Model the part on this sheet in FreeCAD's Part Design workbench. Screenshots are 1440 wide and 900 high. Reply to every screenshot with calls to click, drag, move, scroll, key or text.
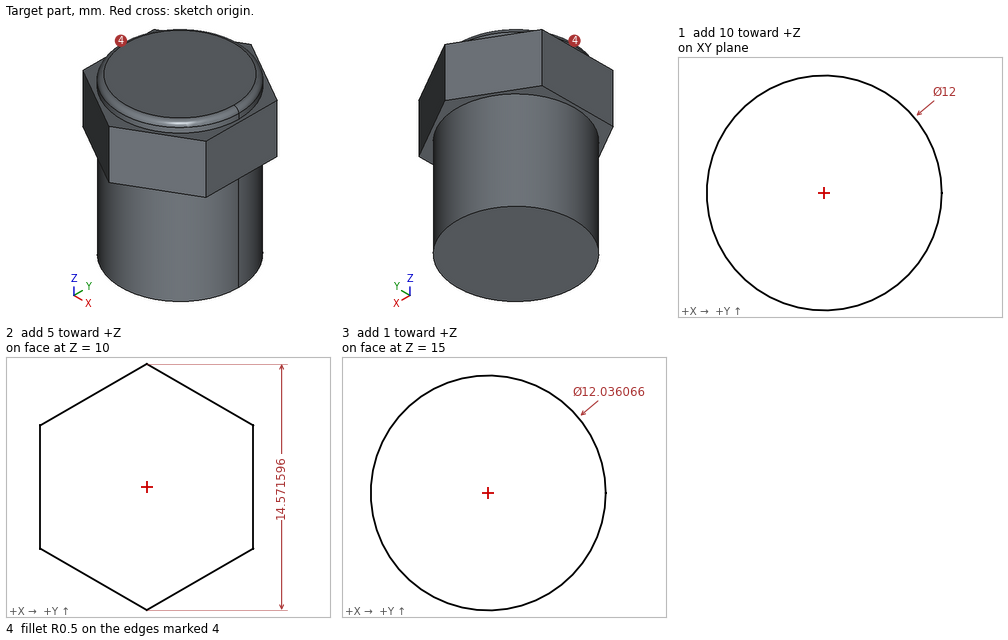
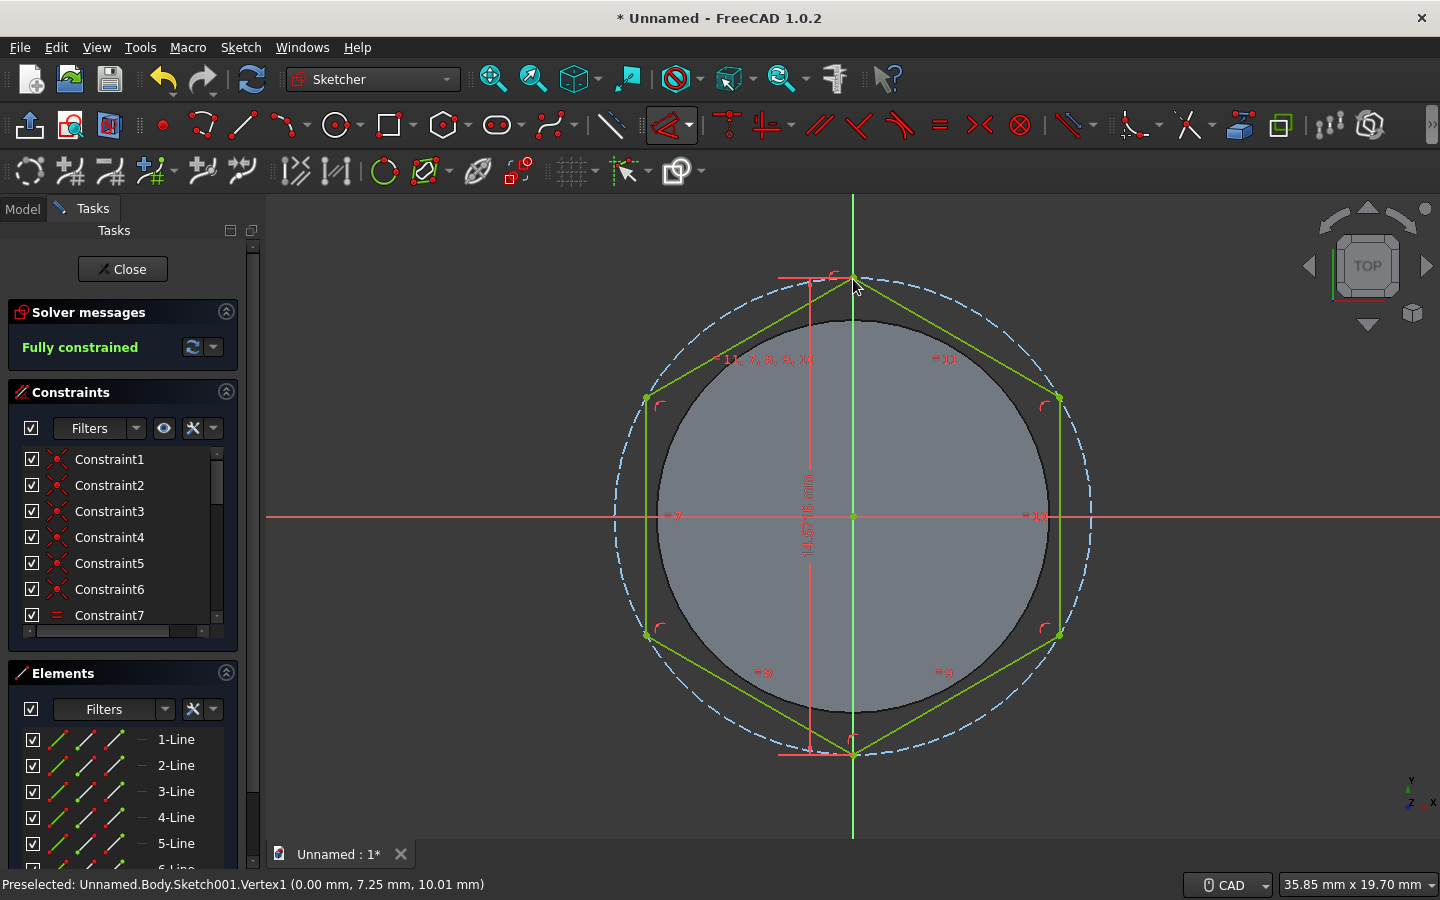
click(123, 269)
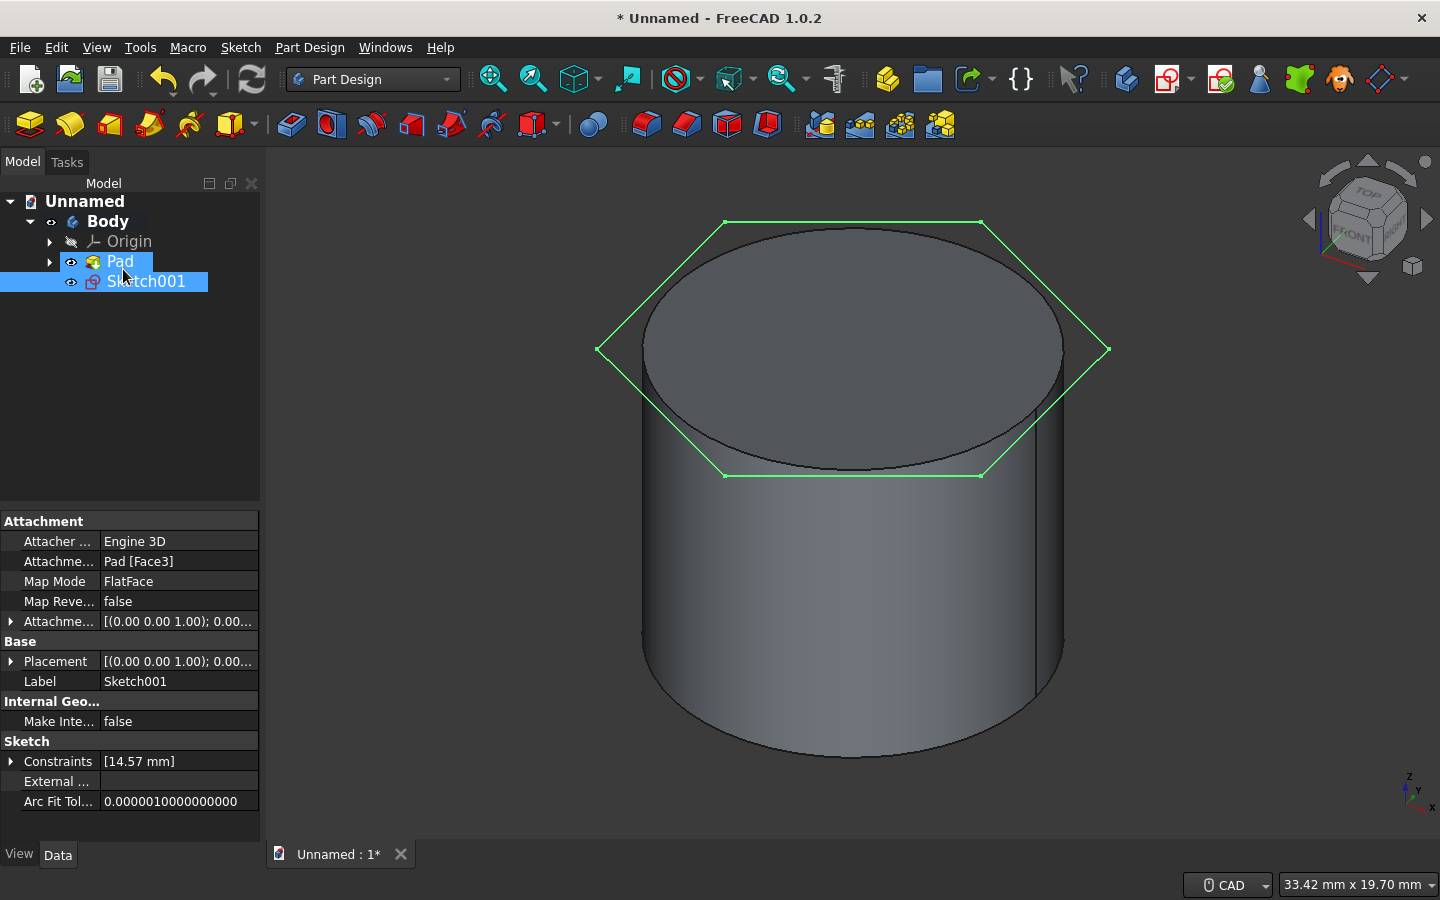
click(30, 124)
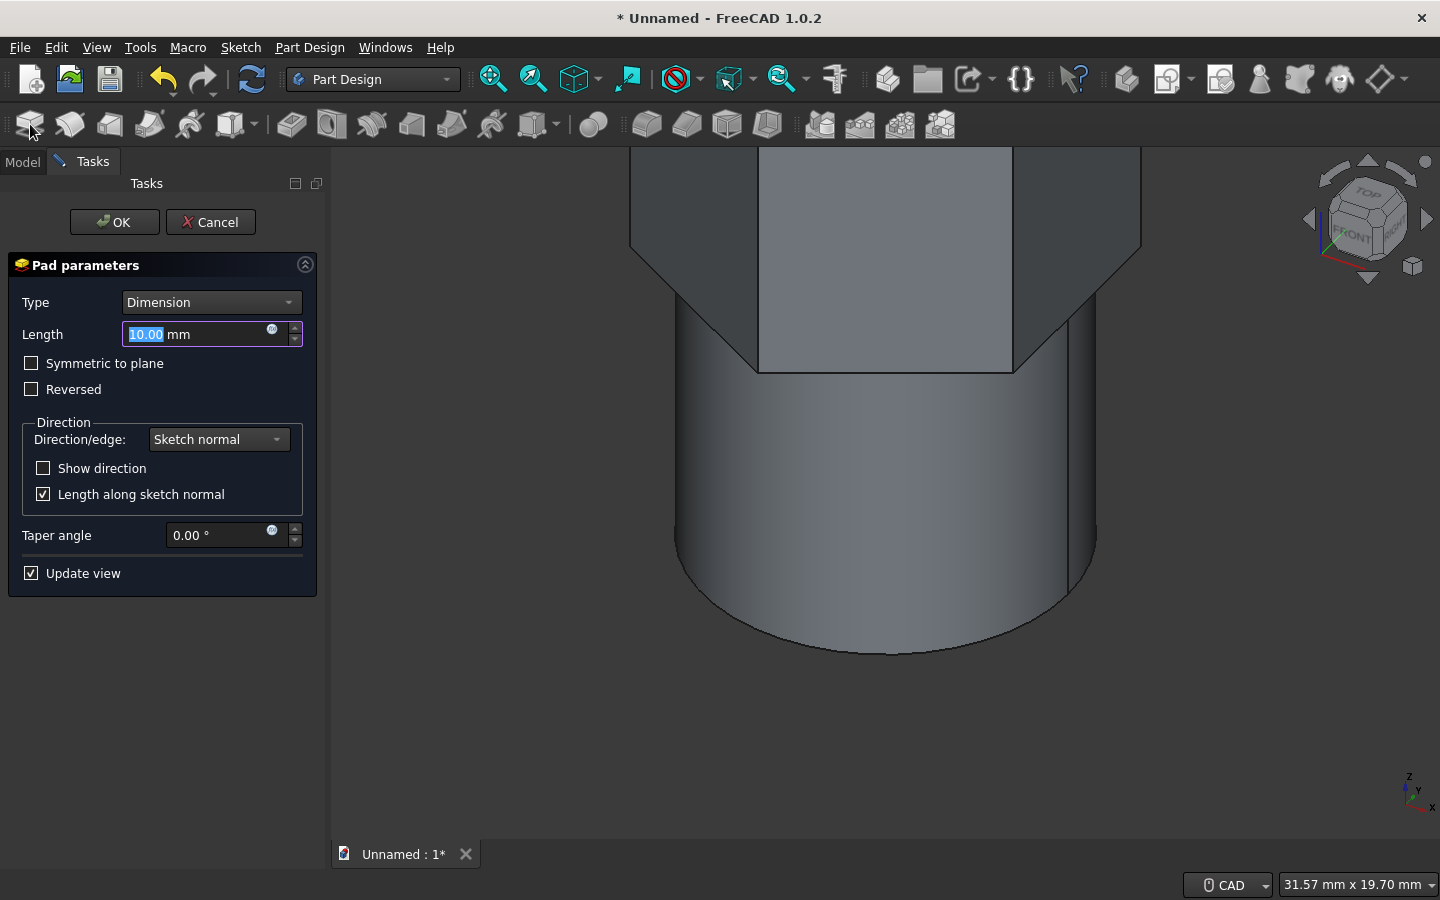
text(5)
key(Tab)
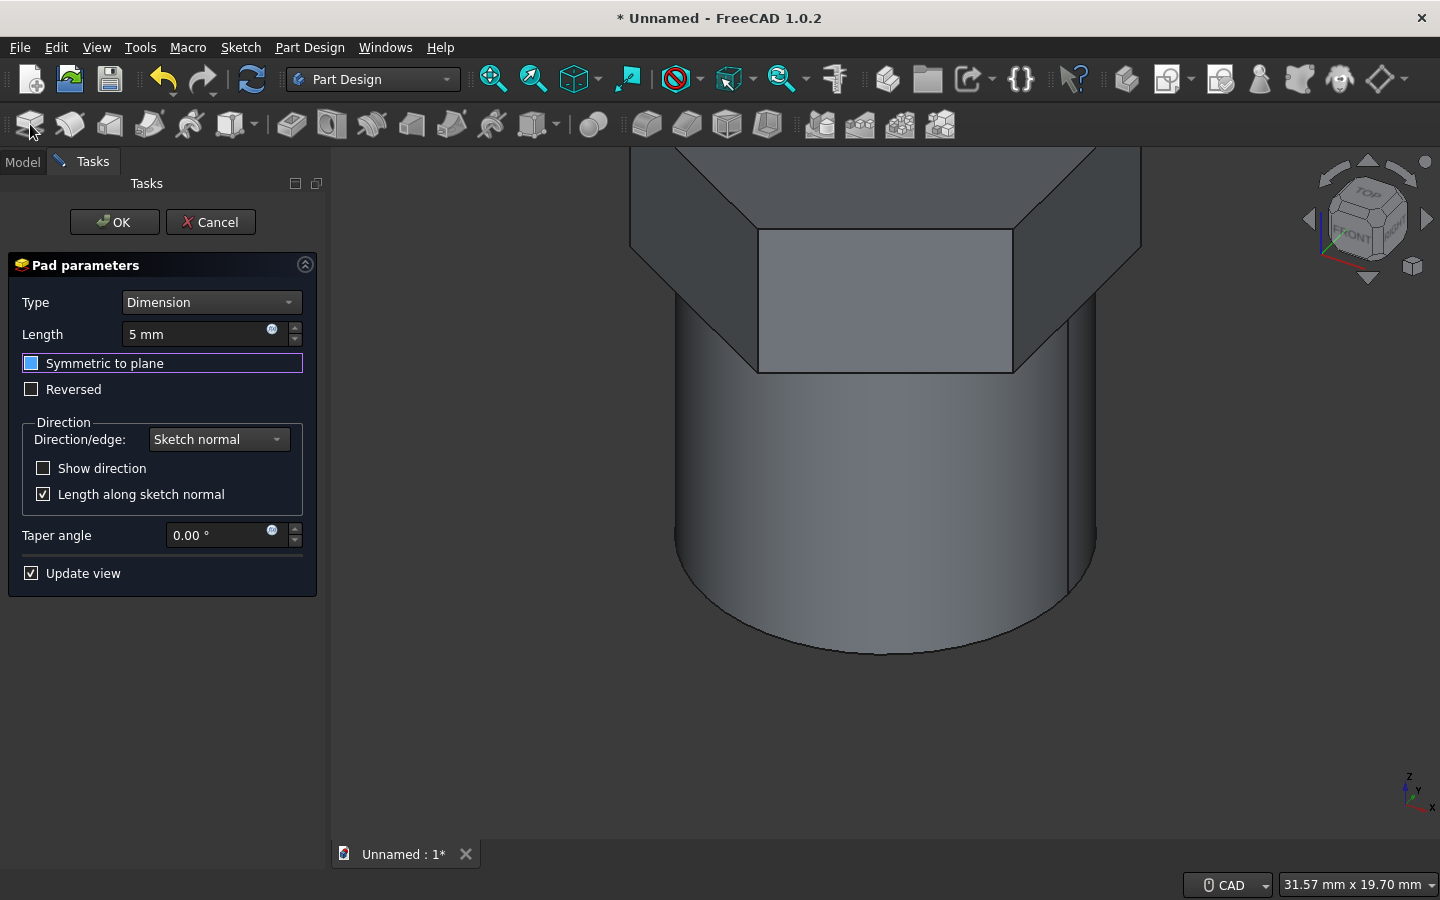
click(115, 222)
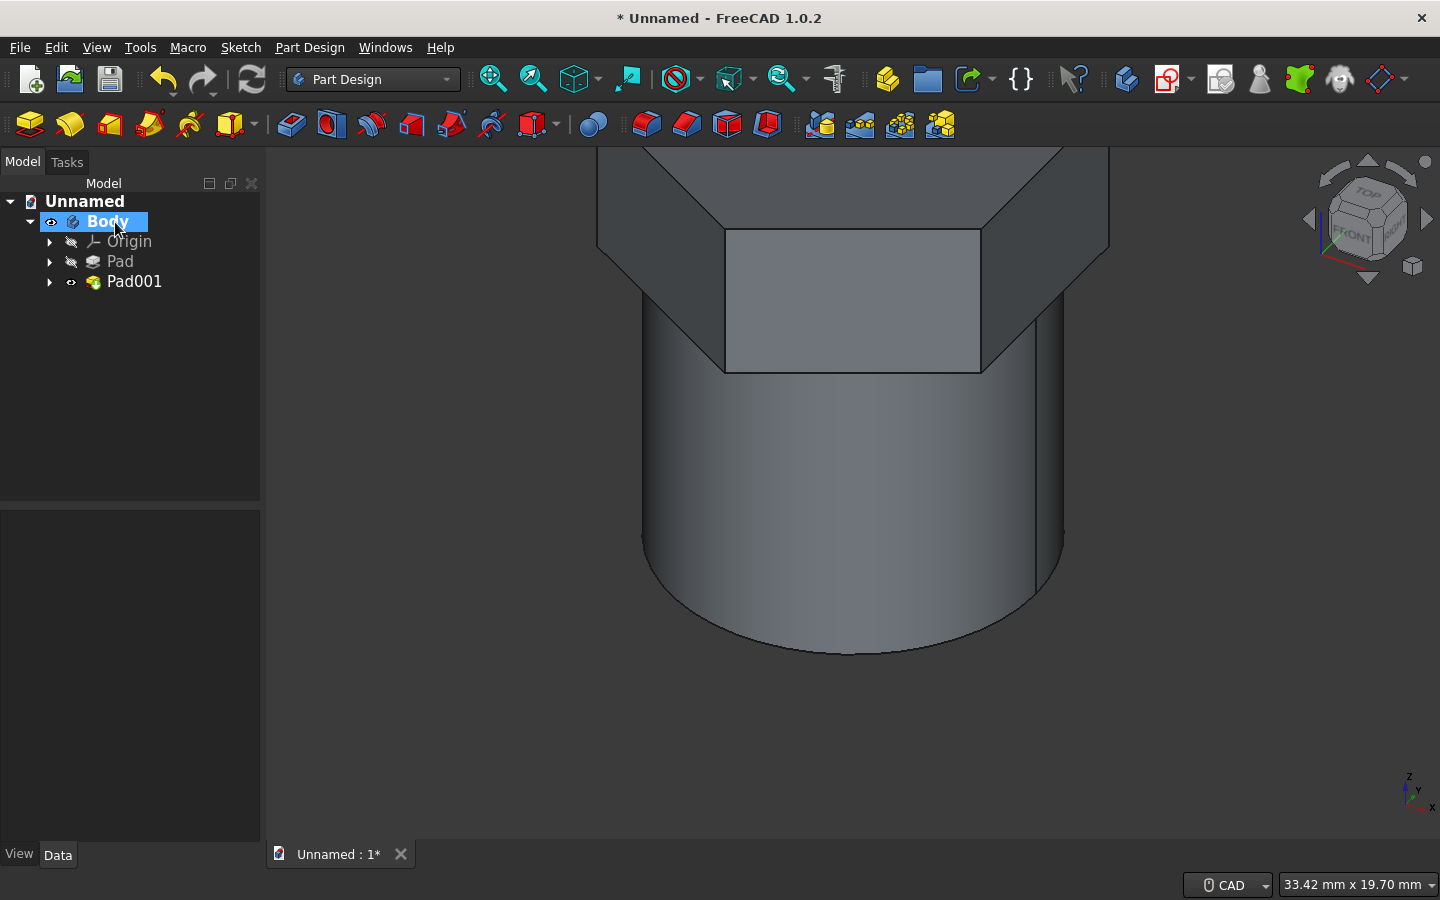
click(494, 80)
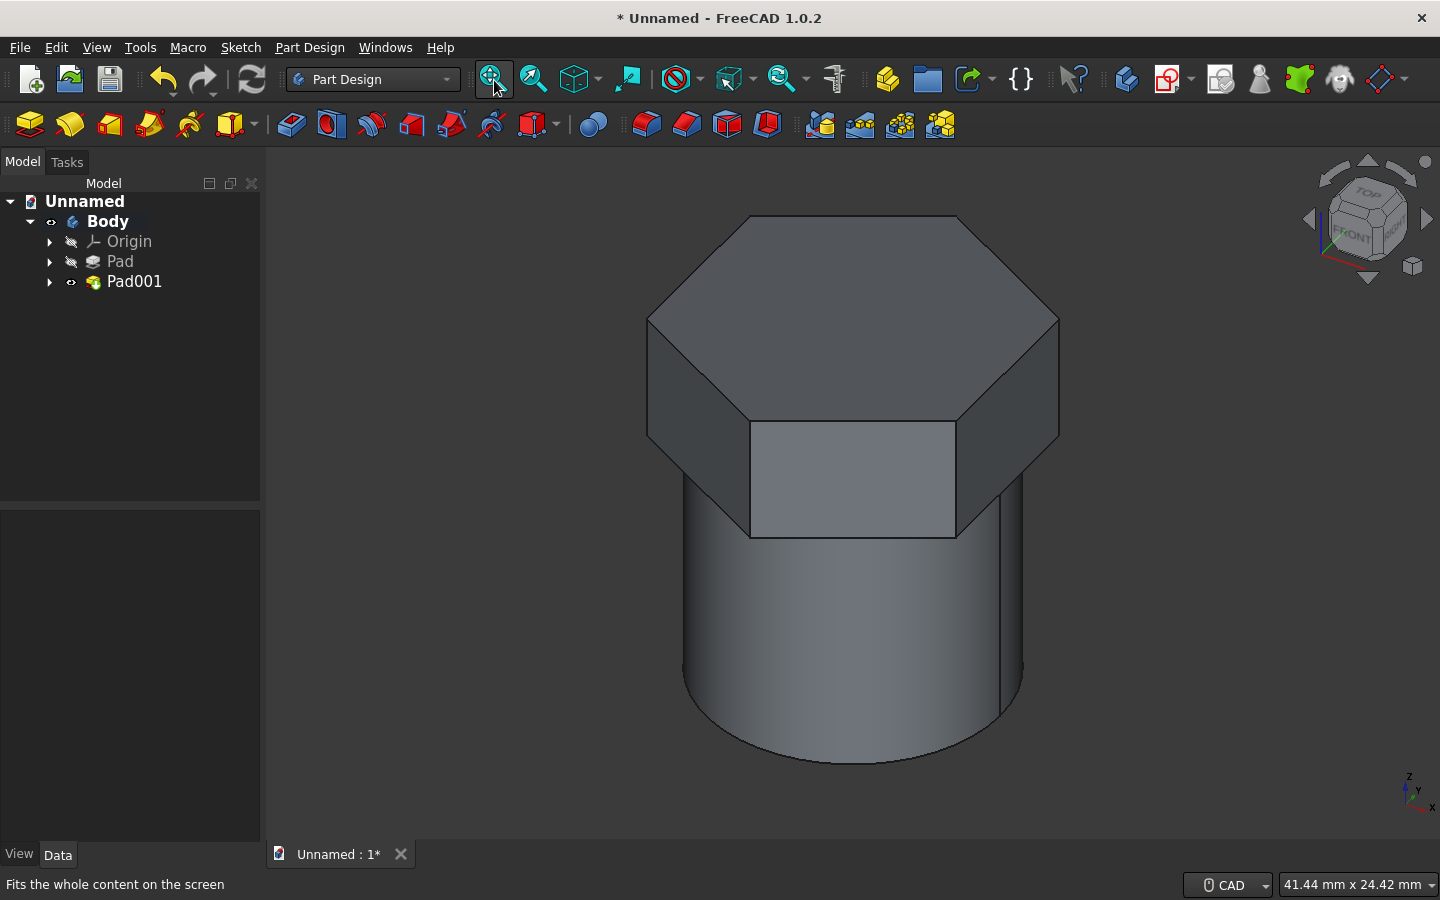
click(853, 318)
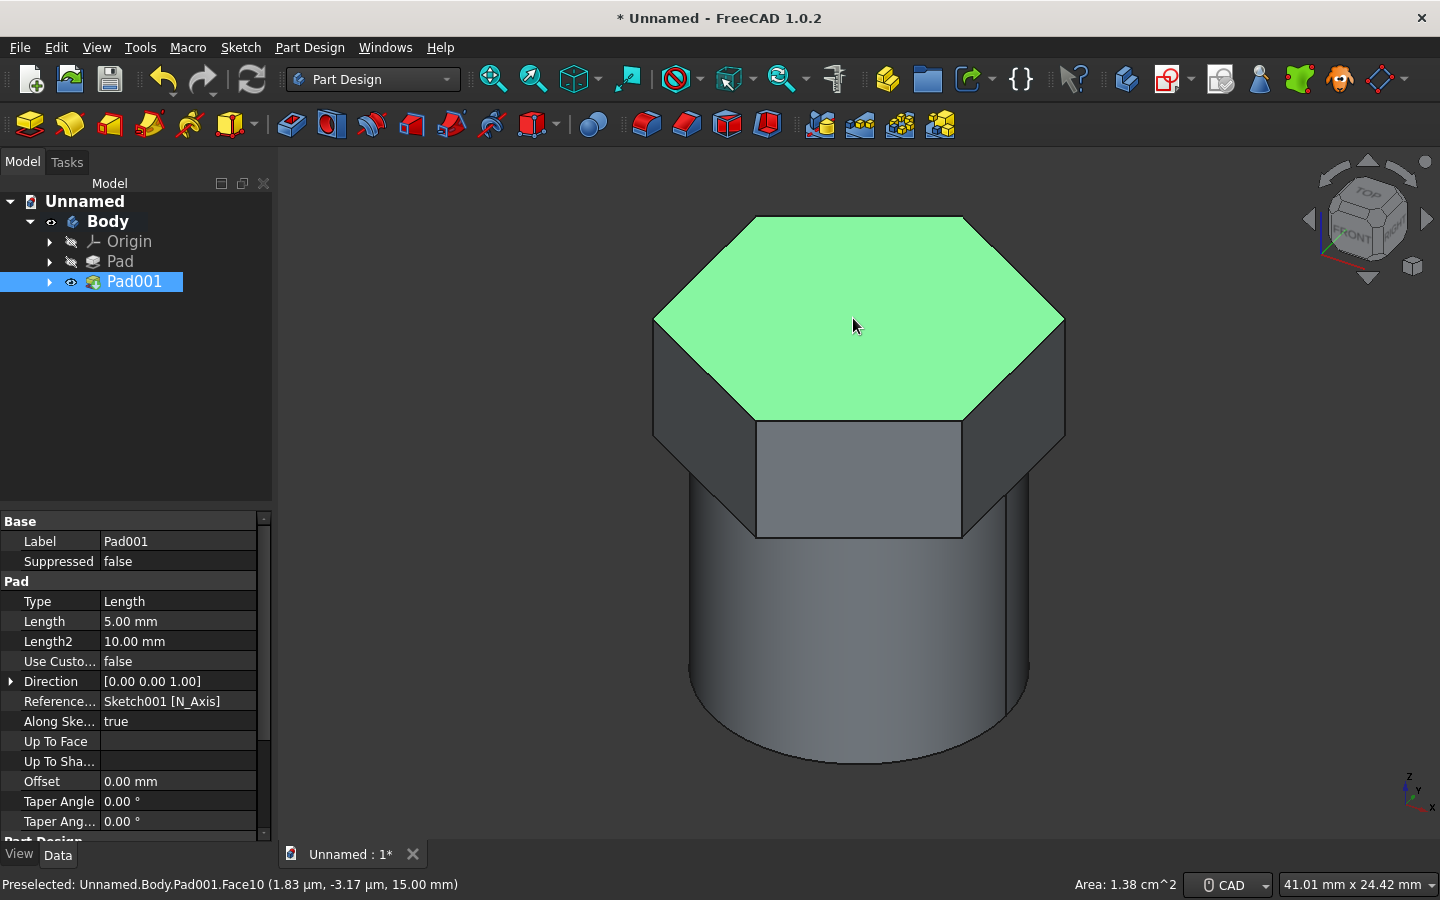
click(1168, 80)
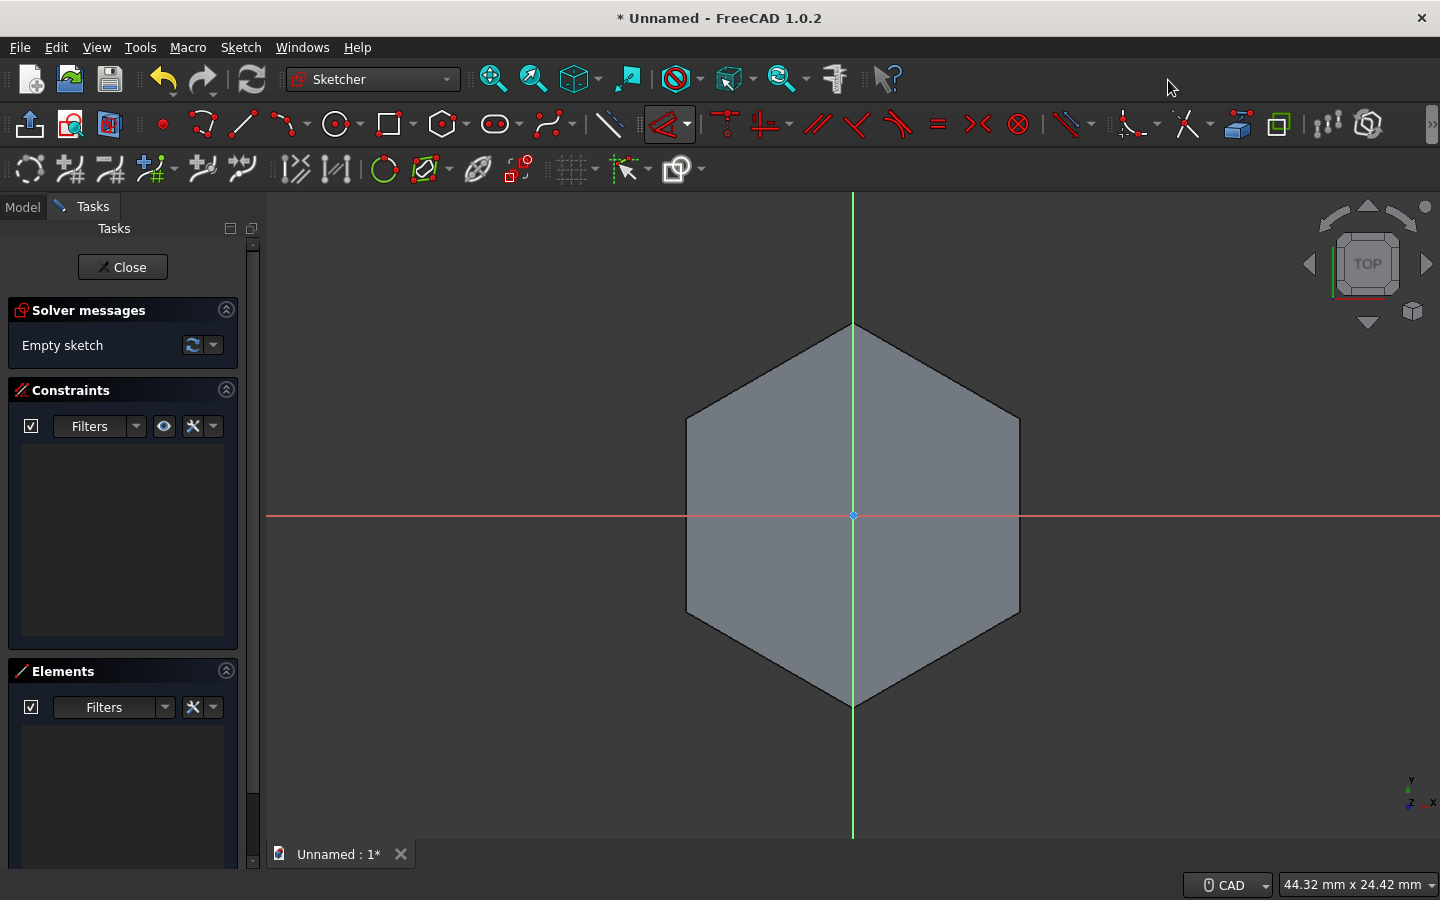
click(336, 124)